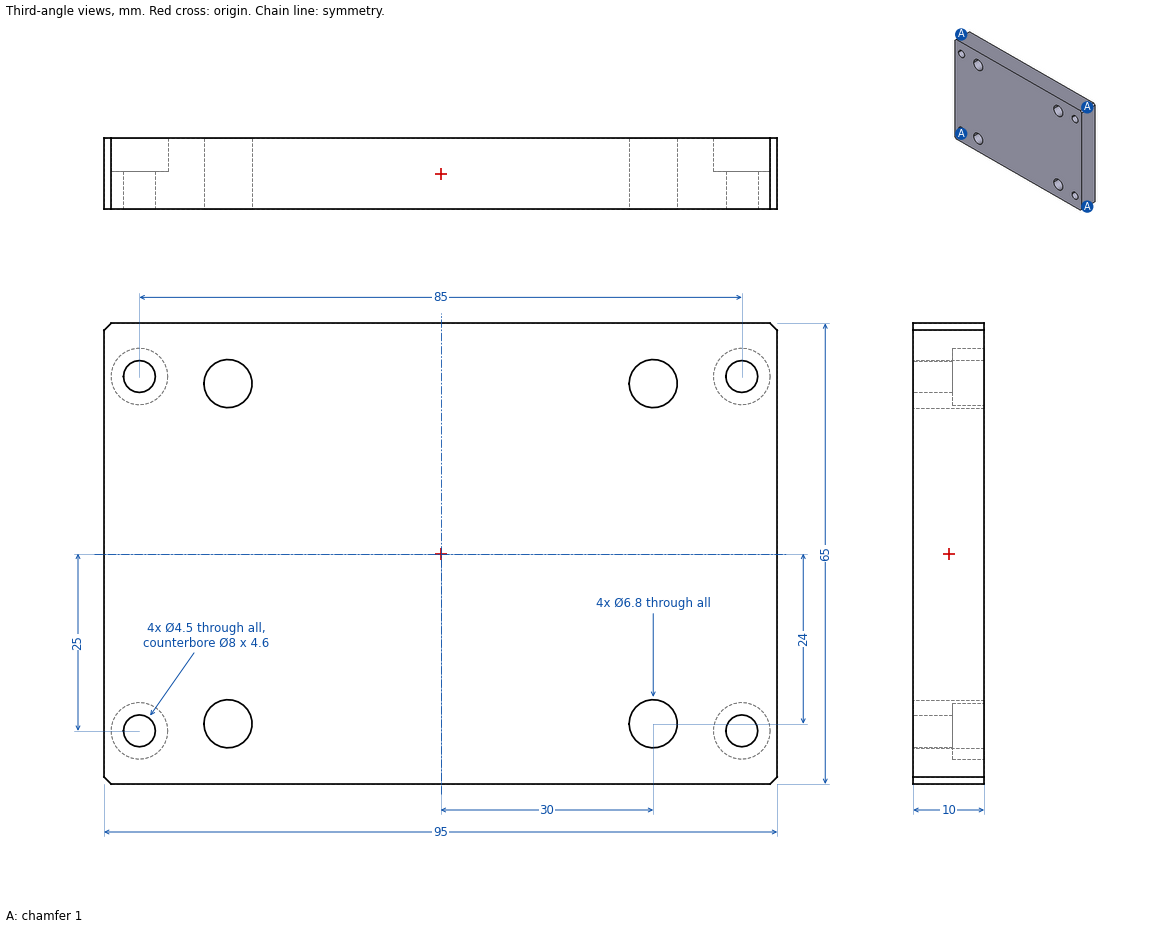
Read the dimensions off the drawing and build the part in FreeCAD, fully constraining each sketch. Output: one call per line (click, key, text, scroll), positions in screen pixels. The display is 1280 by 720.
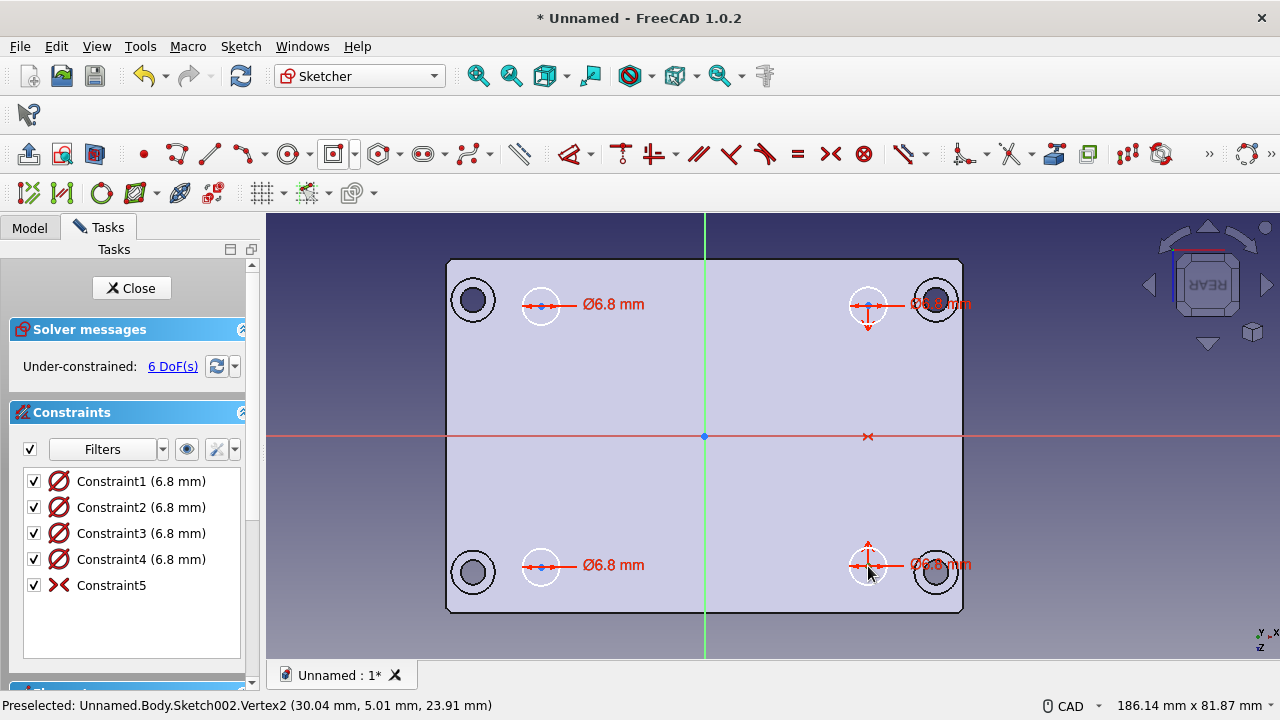
click(541, 567)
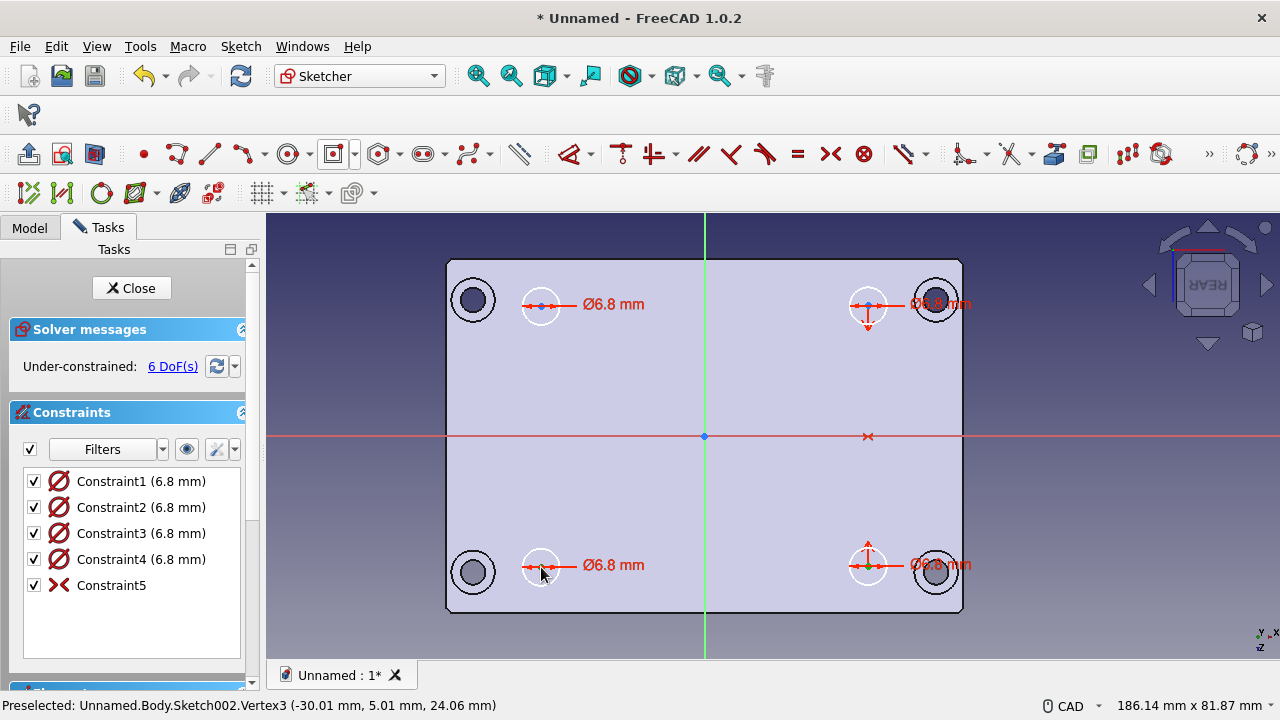
click(705, 603)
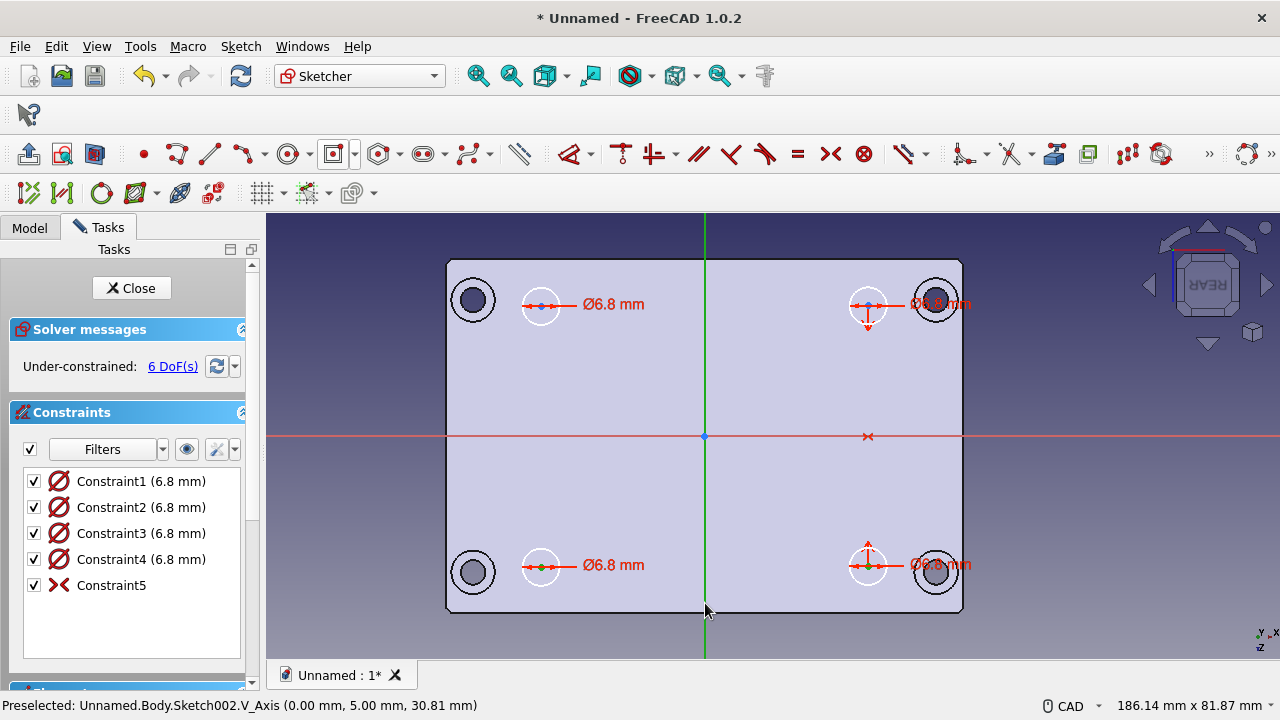
click(831, 154)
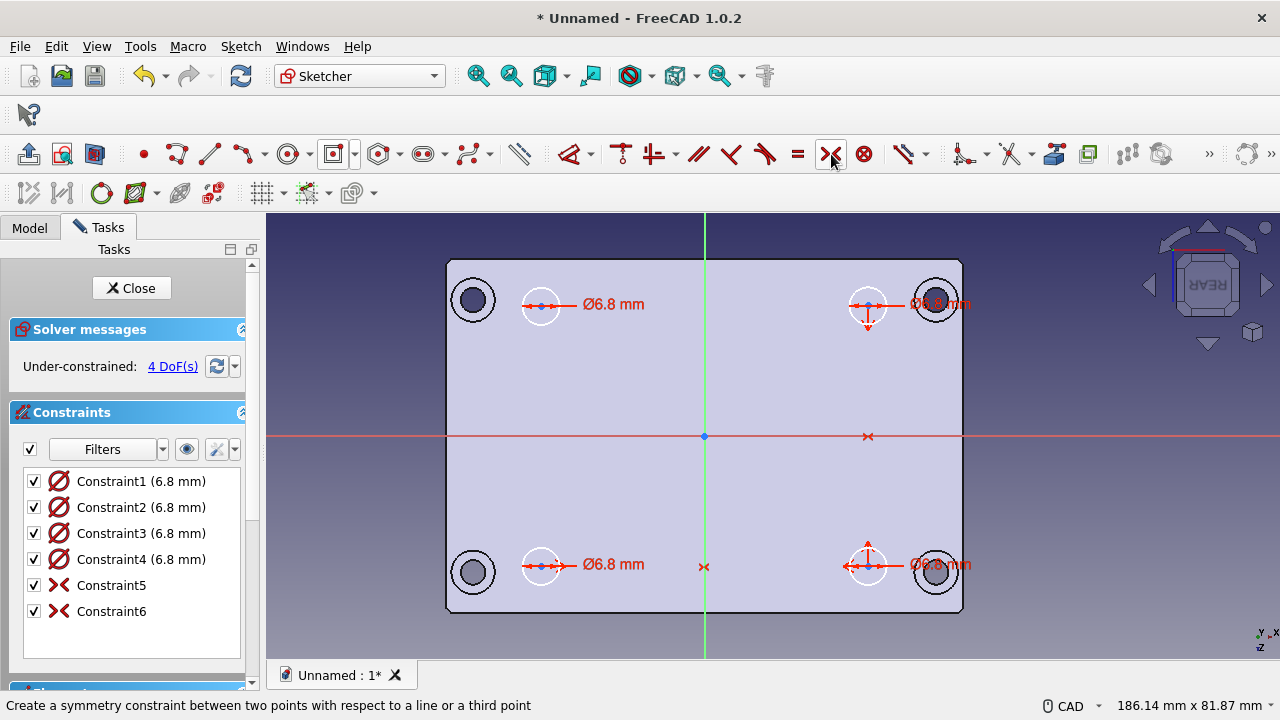
click(868, 306)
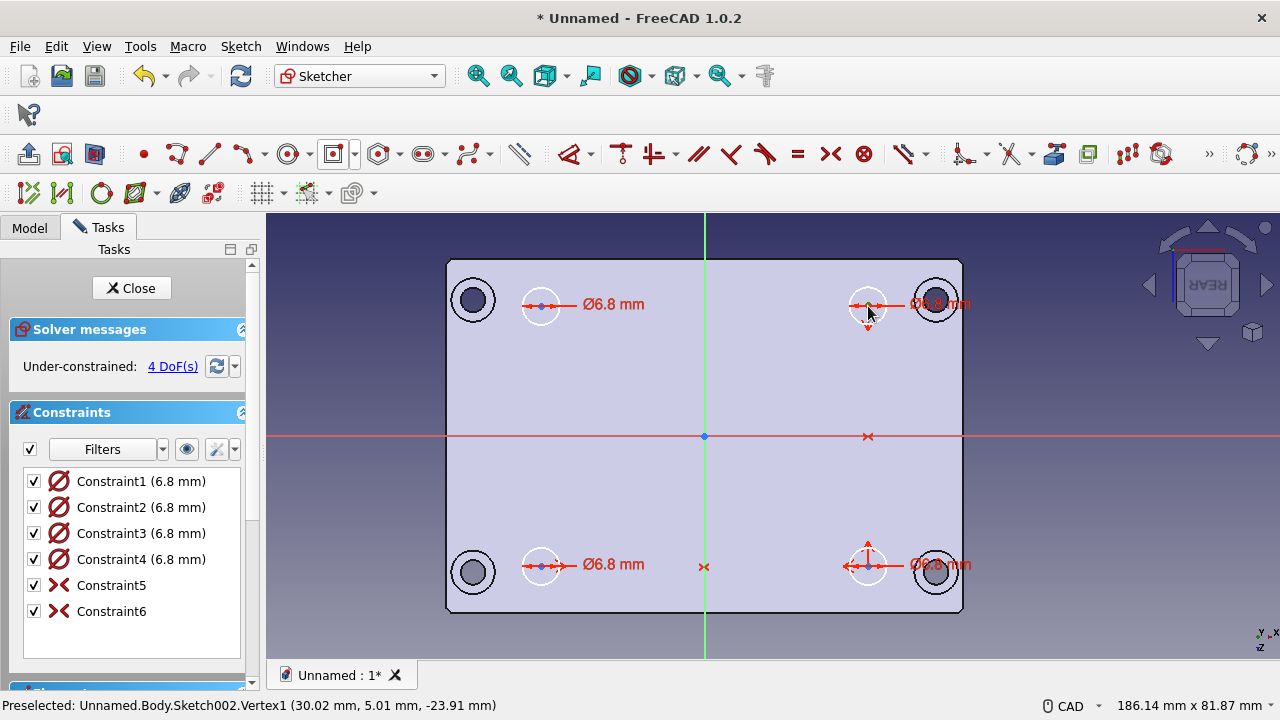
click(541, 306)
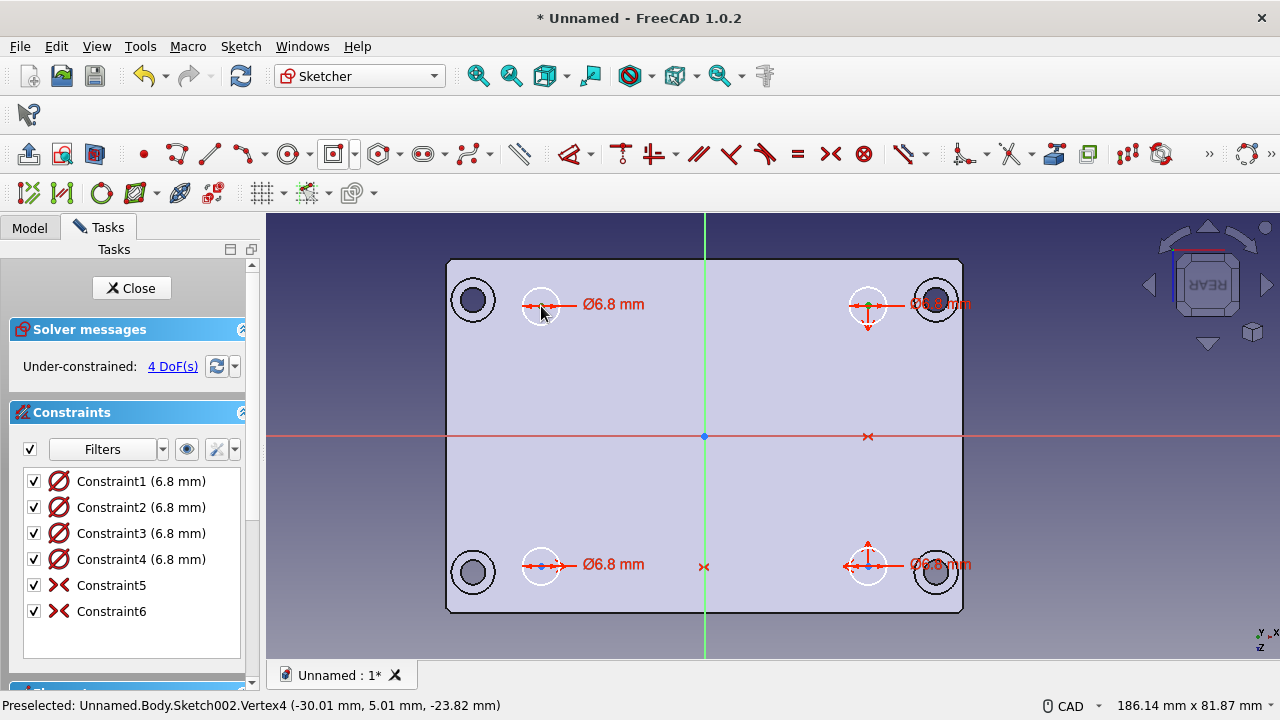
click(705, 603)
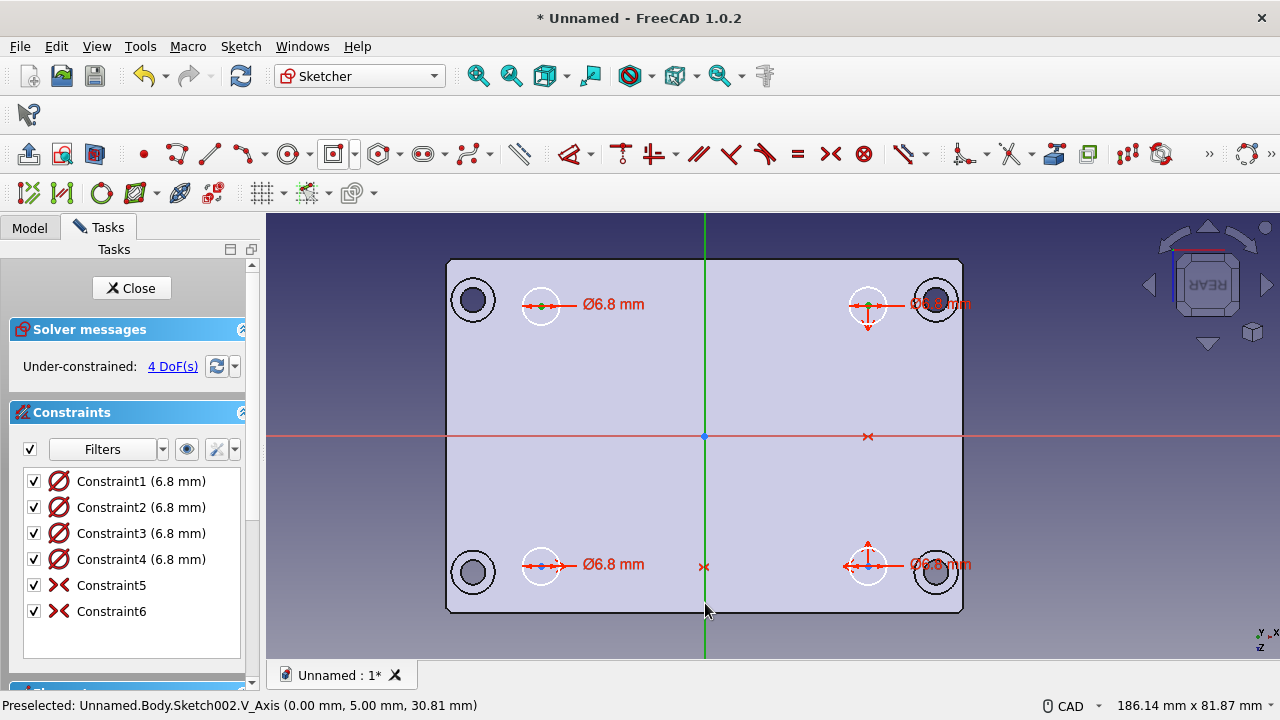
click(831, 154)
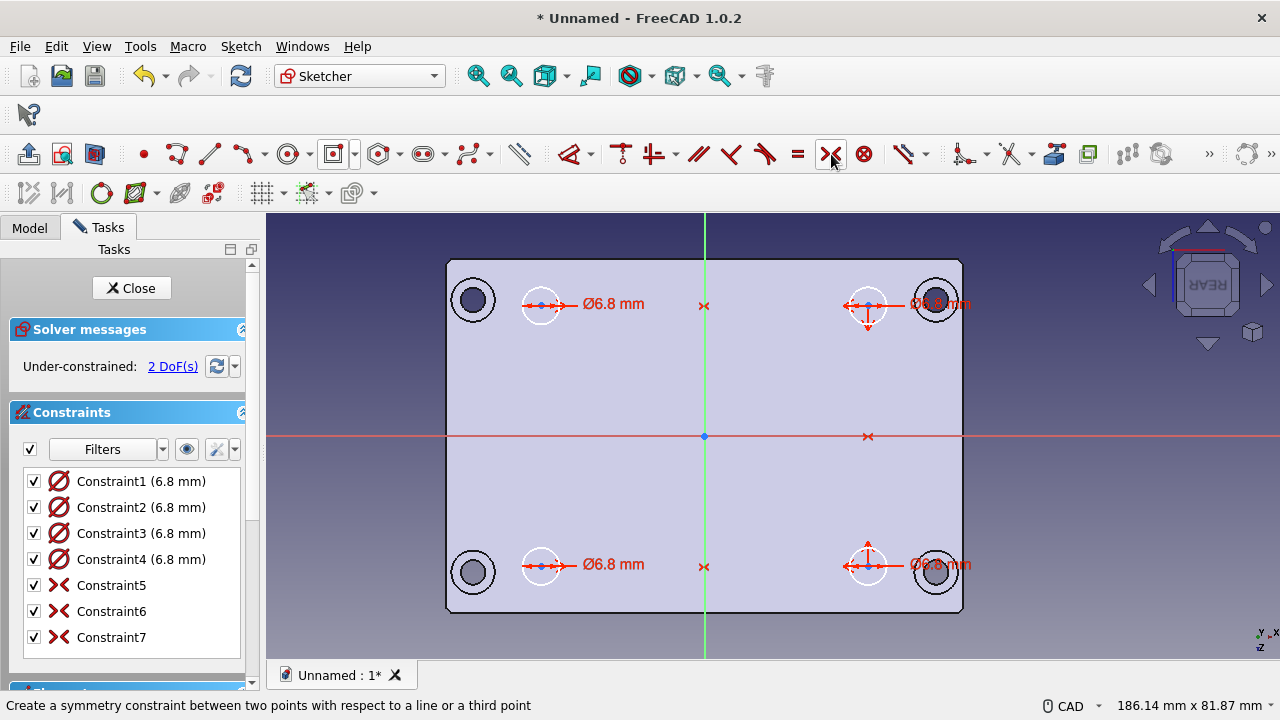
click(568, 154)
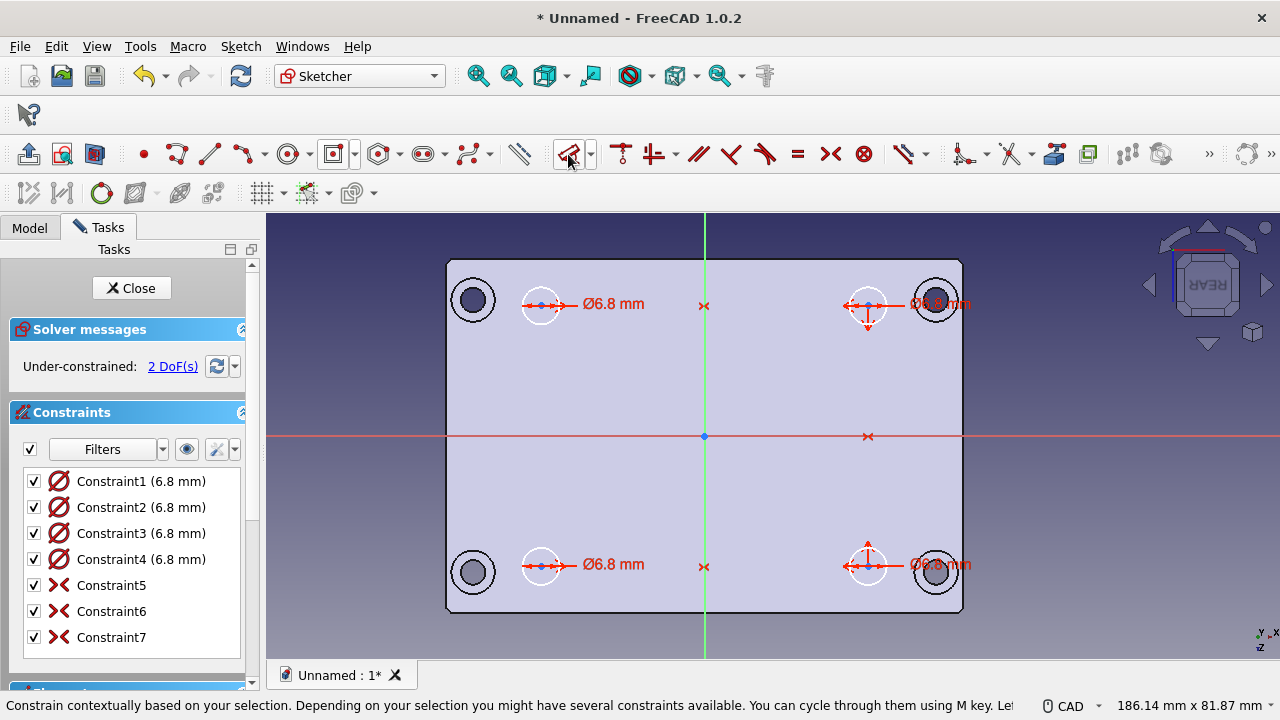
click(868, 306)
click(786, 272)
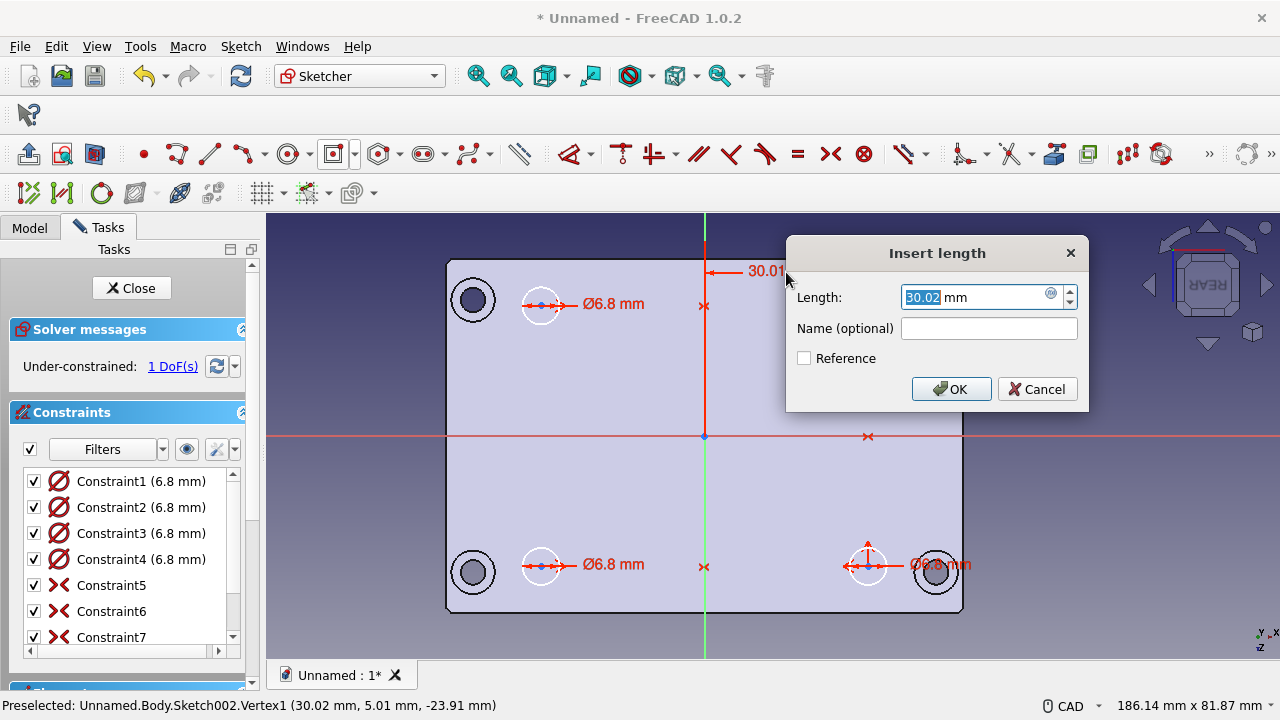
text(30)
key(Return)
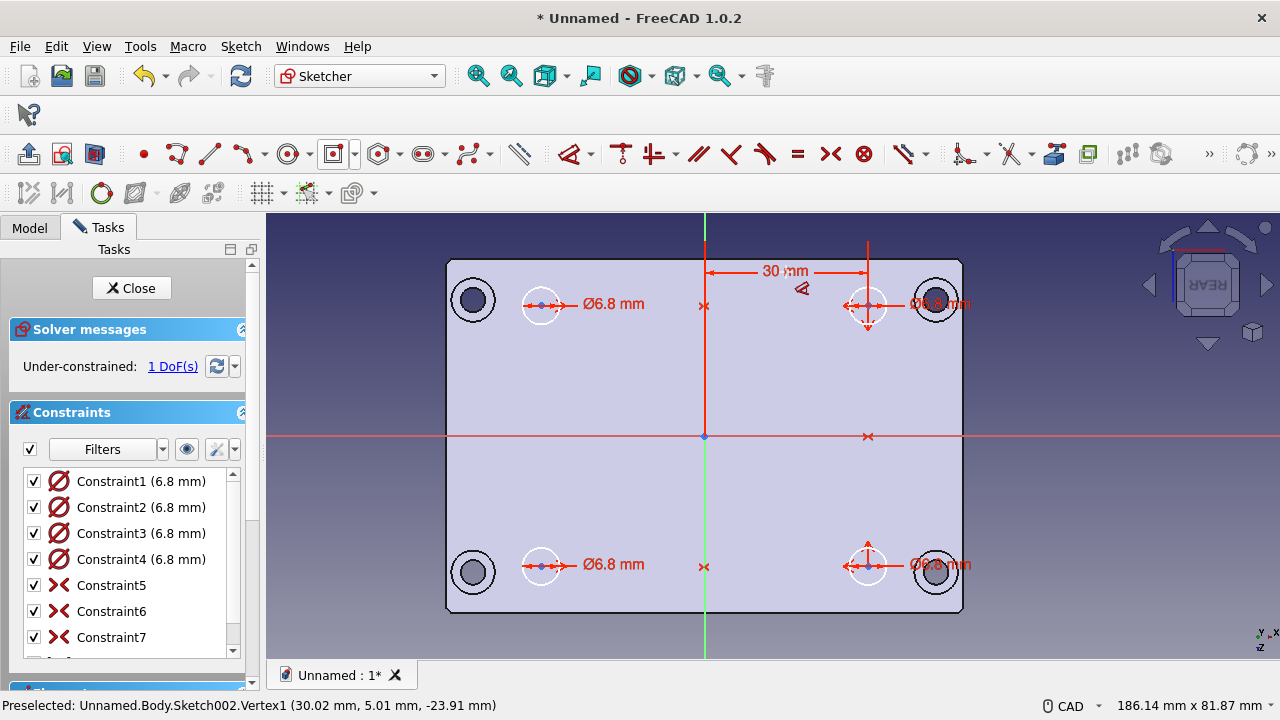
click(868, 306)
click(902, 371)